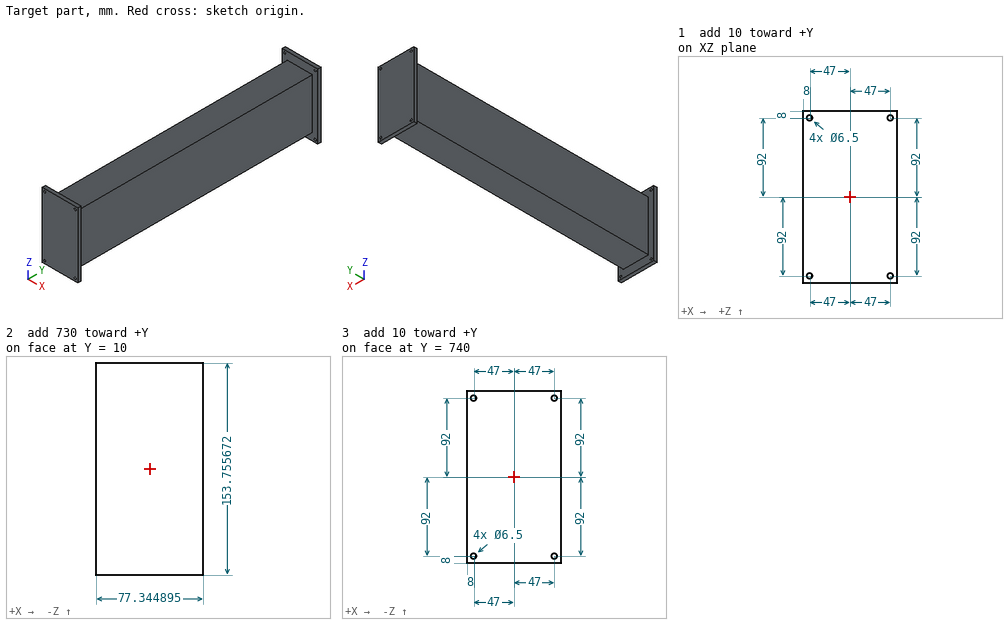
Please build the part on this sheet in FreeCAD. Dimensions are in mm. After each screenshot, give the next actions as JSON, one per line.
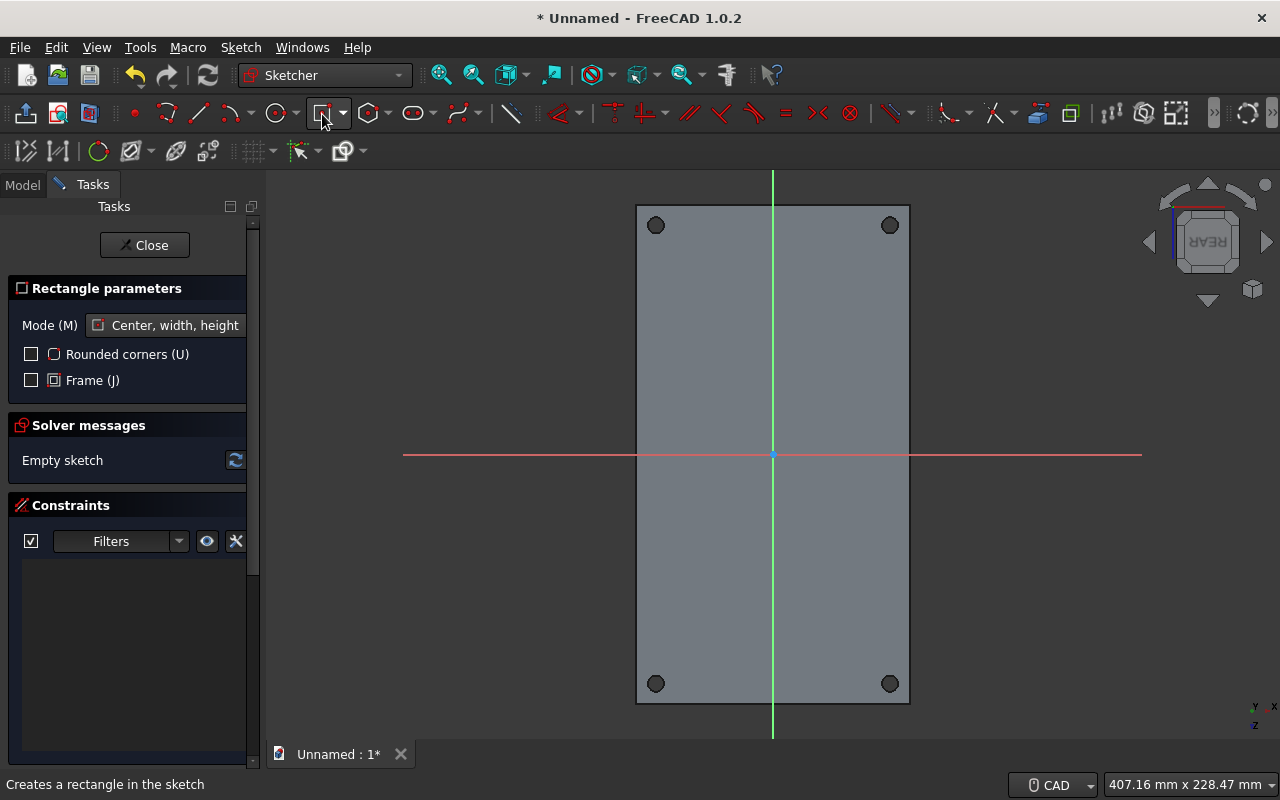
{"action": "left_click", "coordinate": [773, 455]}
{"action": "left_click", "coordinate": [869, 263]}
{"action": "key", "text": "Escape"}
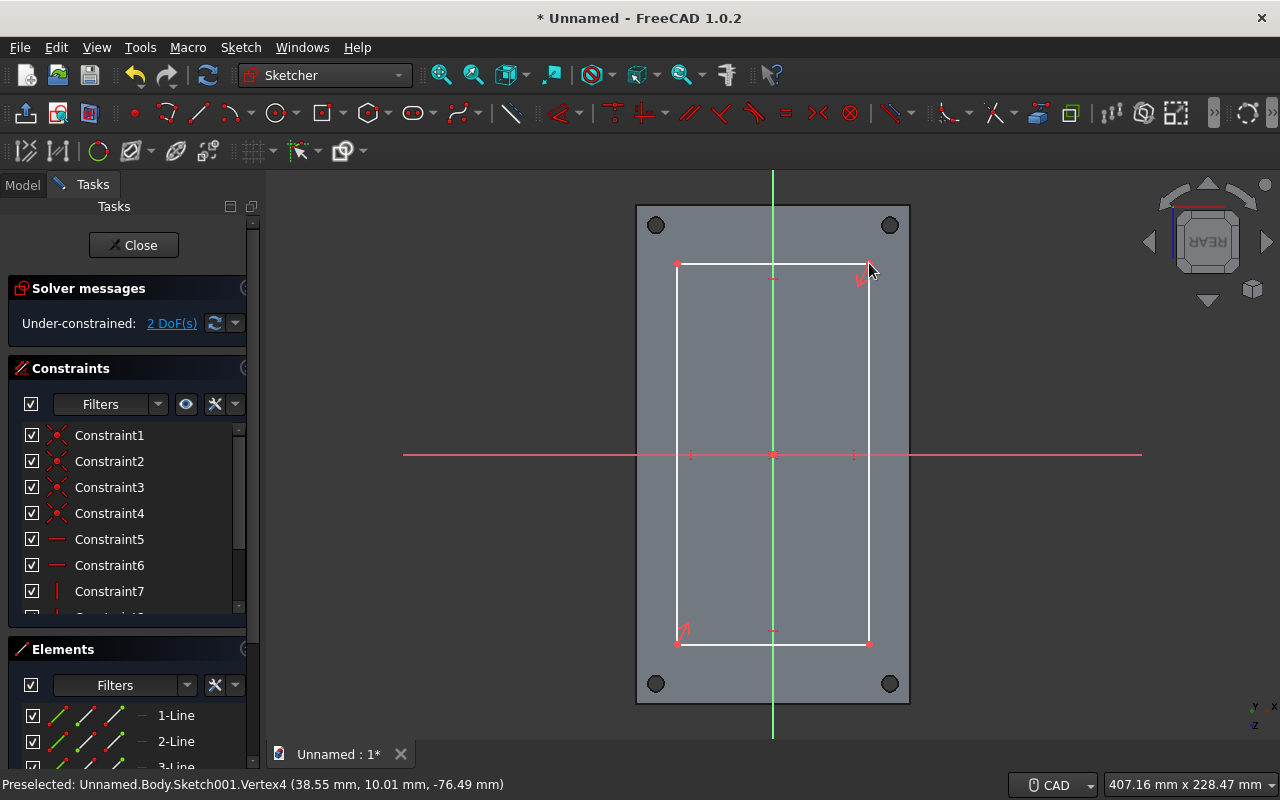
{"action": "left_click", "coordinate": [558, 114]}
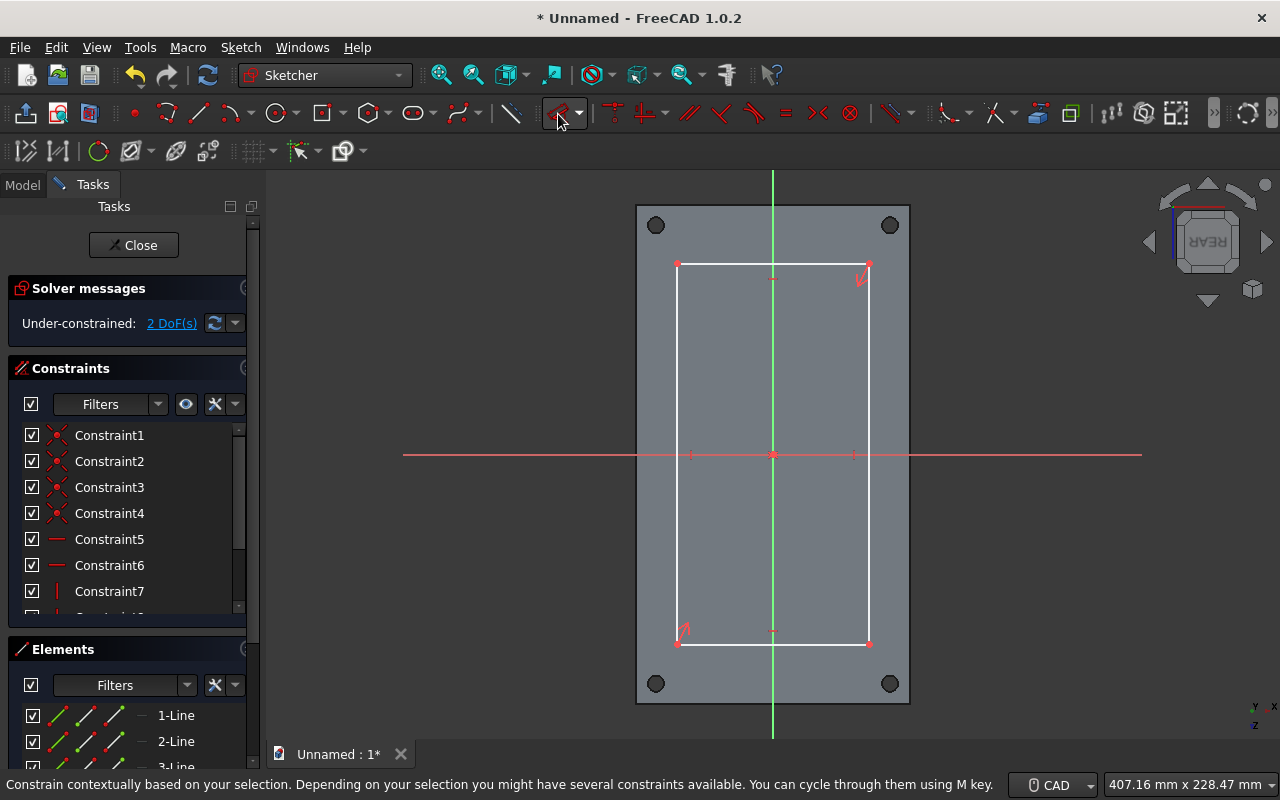
{"action": "left_click", "coordinate": [735, 645]}
{"action": "left_click", "coordinate": [729, 679]}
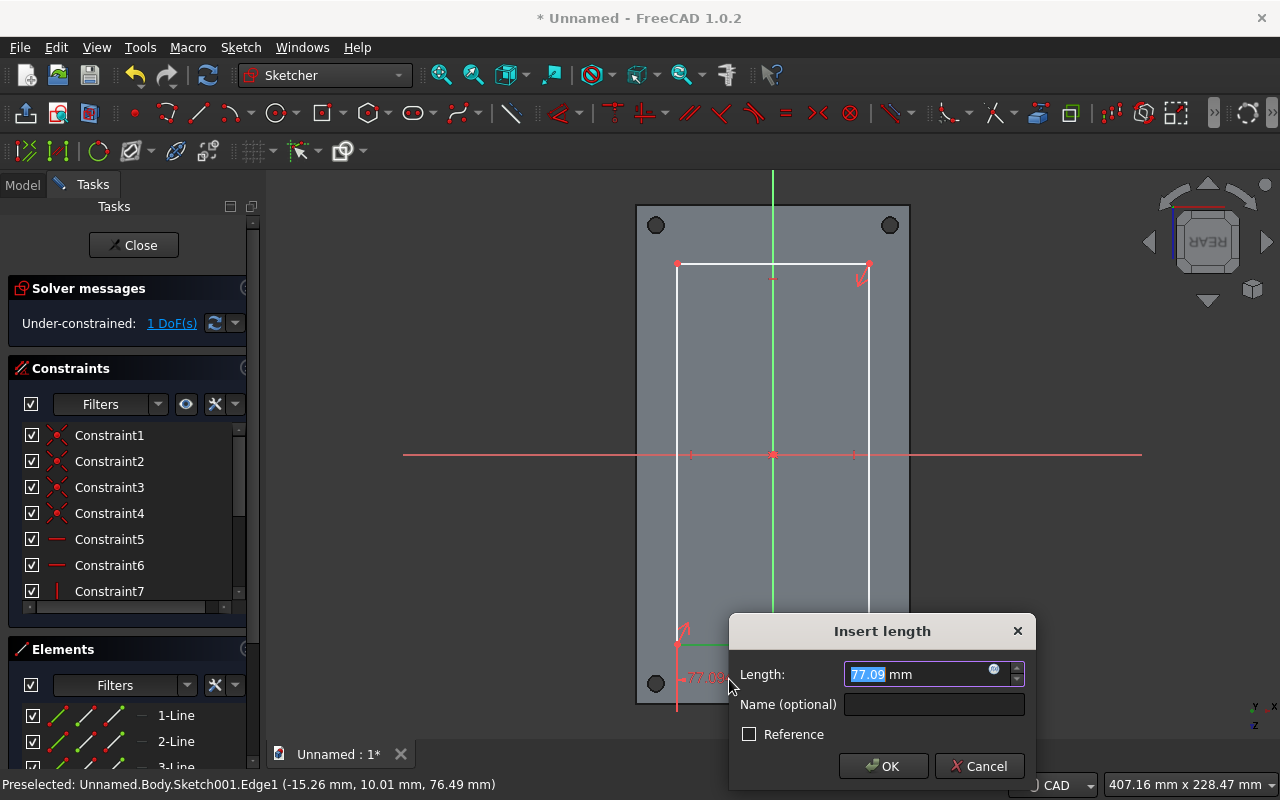
{"action": "type", "text": "77.344895"}
{"action": "key", "text": "Return"}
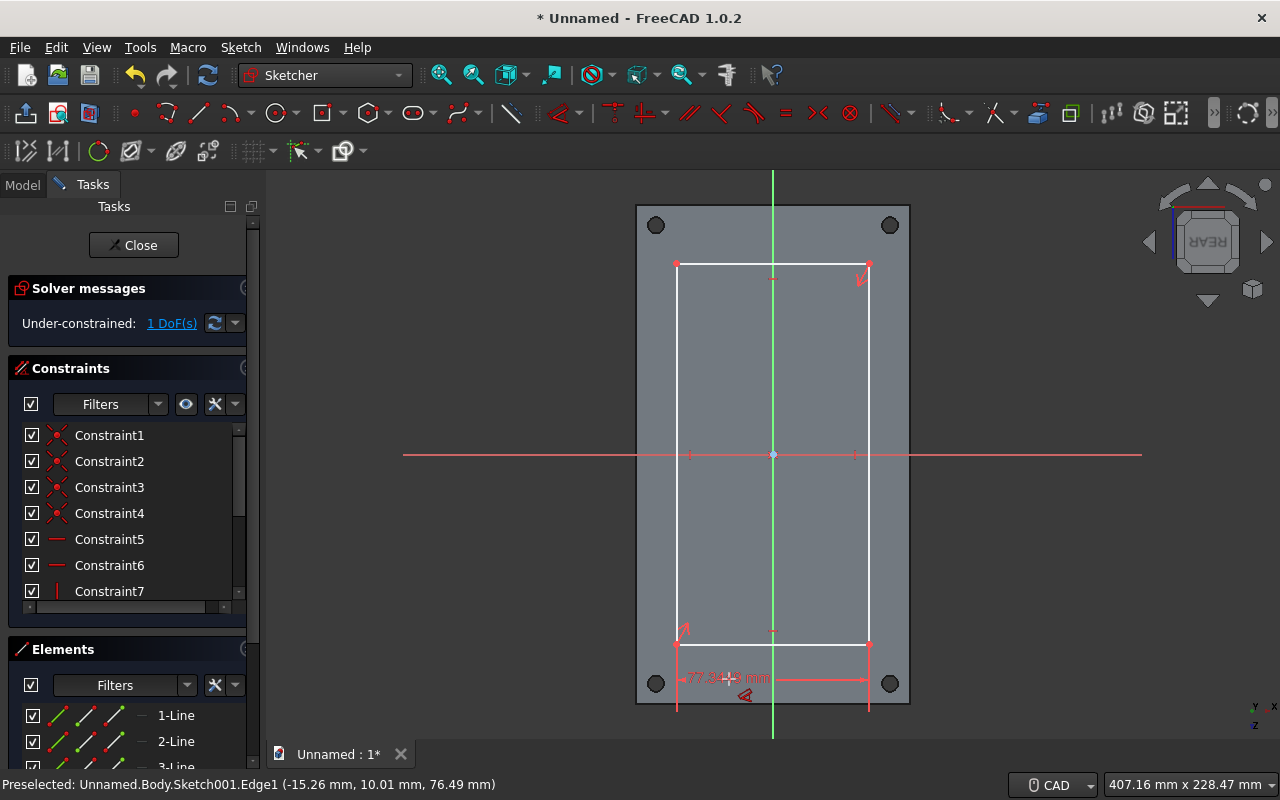
{"action": "left_click", "coordinate": [869, 531]}
{"action": "left_click", "coordinate": [903, 367]}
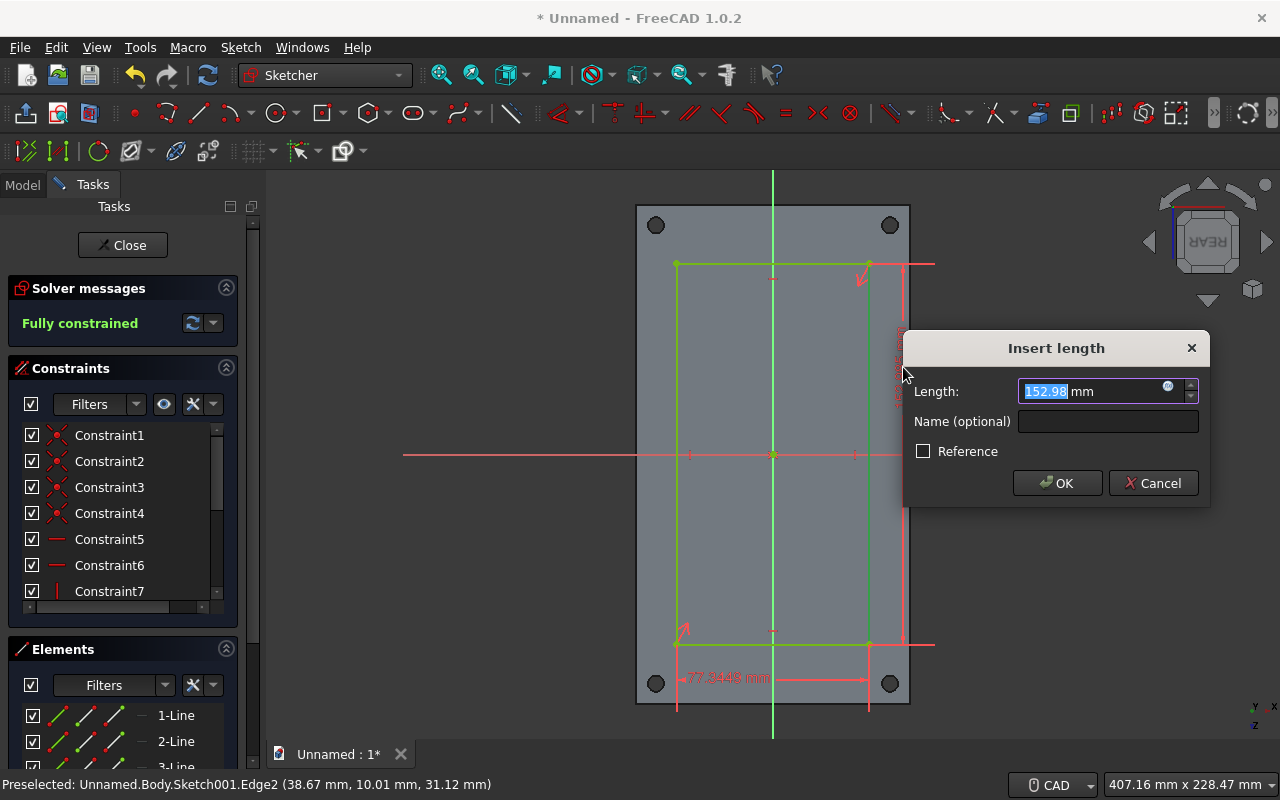
{"action": "type", "text": "153.755672"}
{"action": "key", "text": "Return"}
{"action": "key", "text": "Escape"}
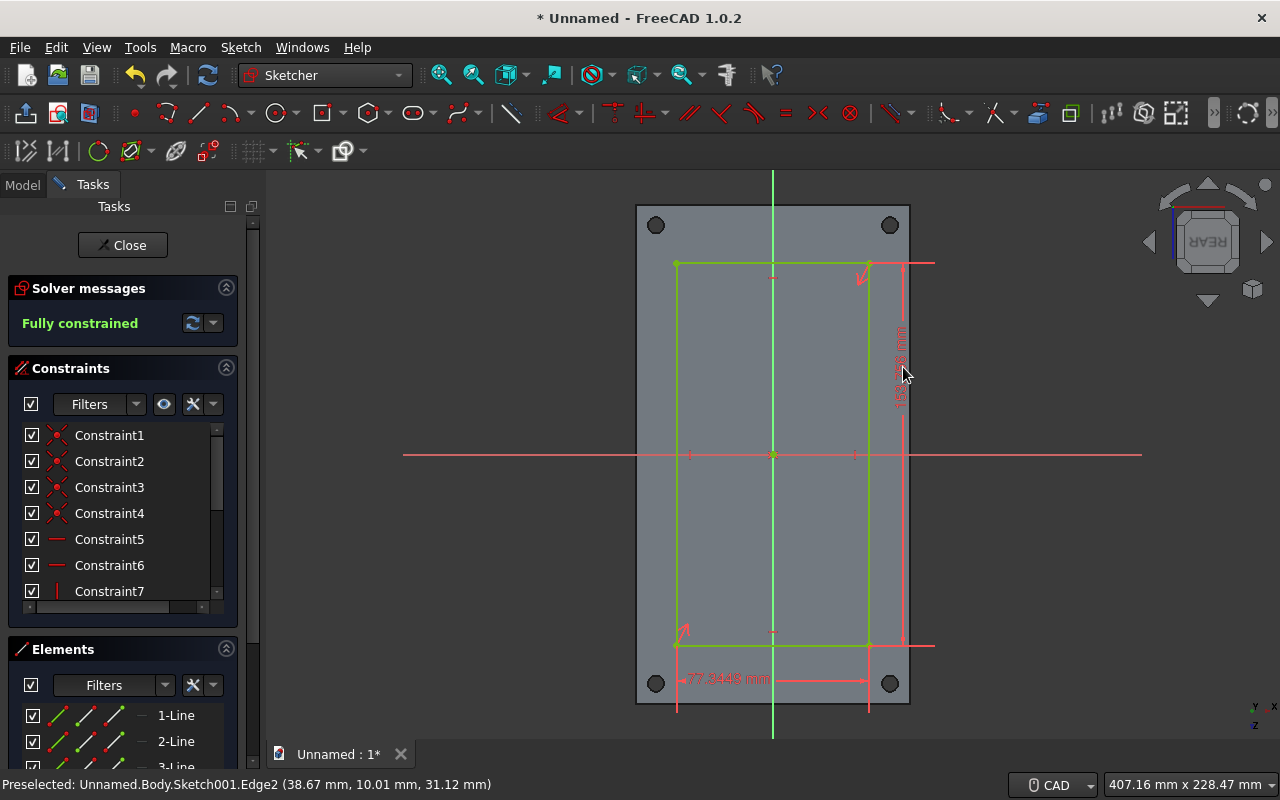
{"action": "left_click", "coordinate": [123, 245]}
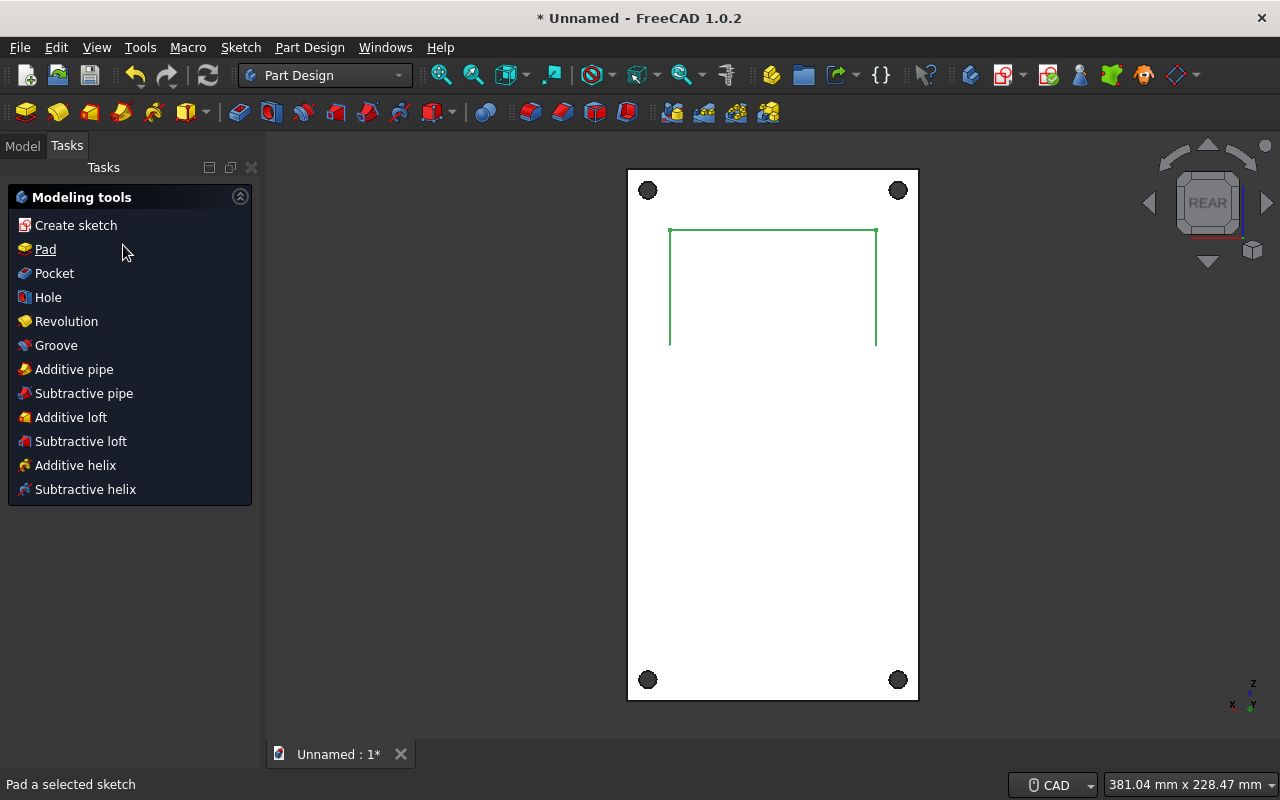
{"action": "left_click", "coordinate": [26, 112]}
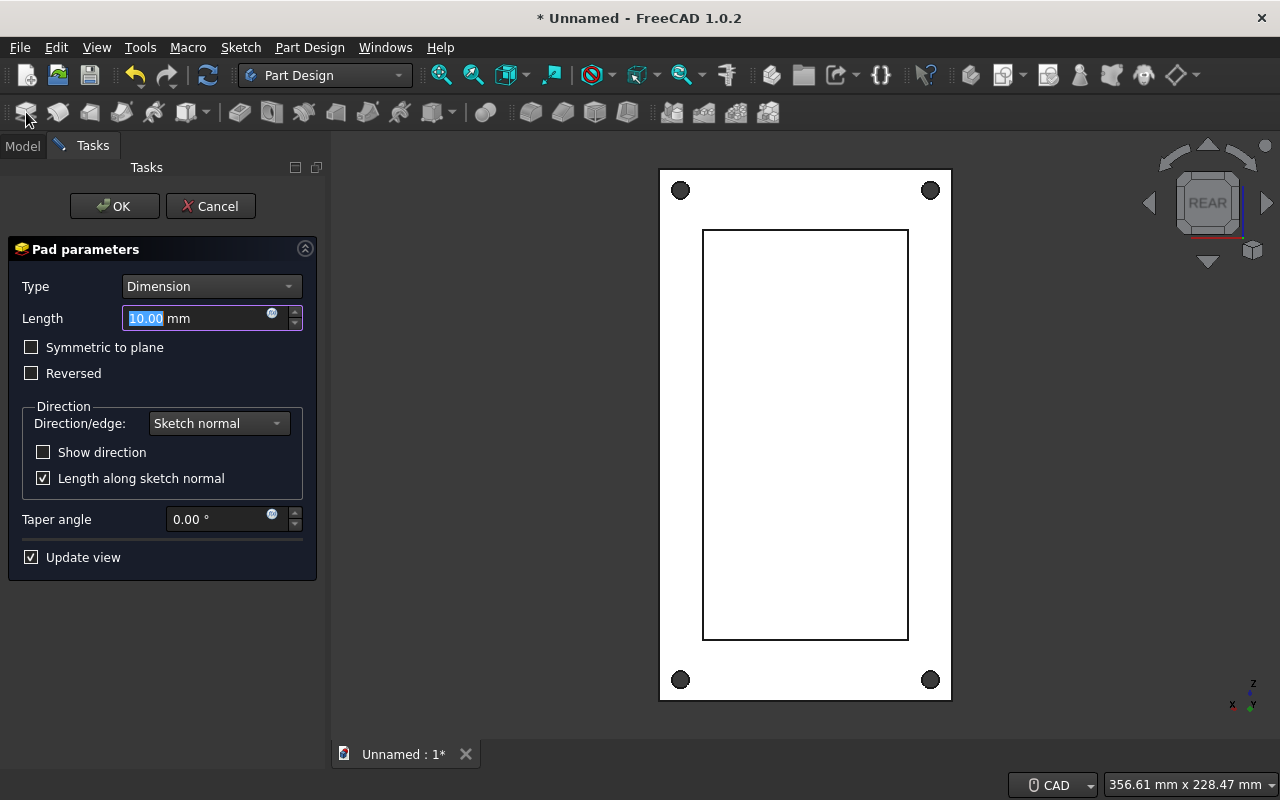
{"action": "type", "text": "730"}
{"action": "key", "text": "Tab"}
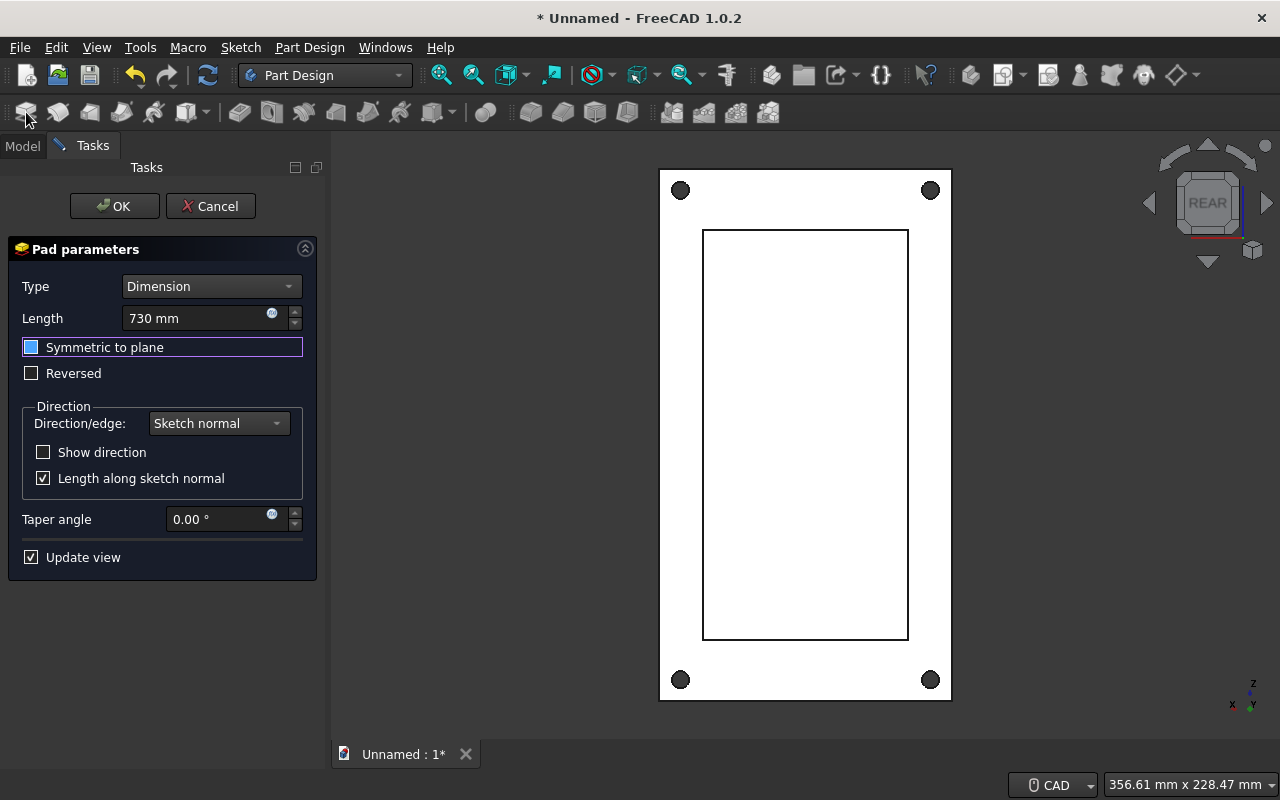
{"action": "left_click", "coordinate": [115, 206]}